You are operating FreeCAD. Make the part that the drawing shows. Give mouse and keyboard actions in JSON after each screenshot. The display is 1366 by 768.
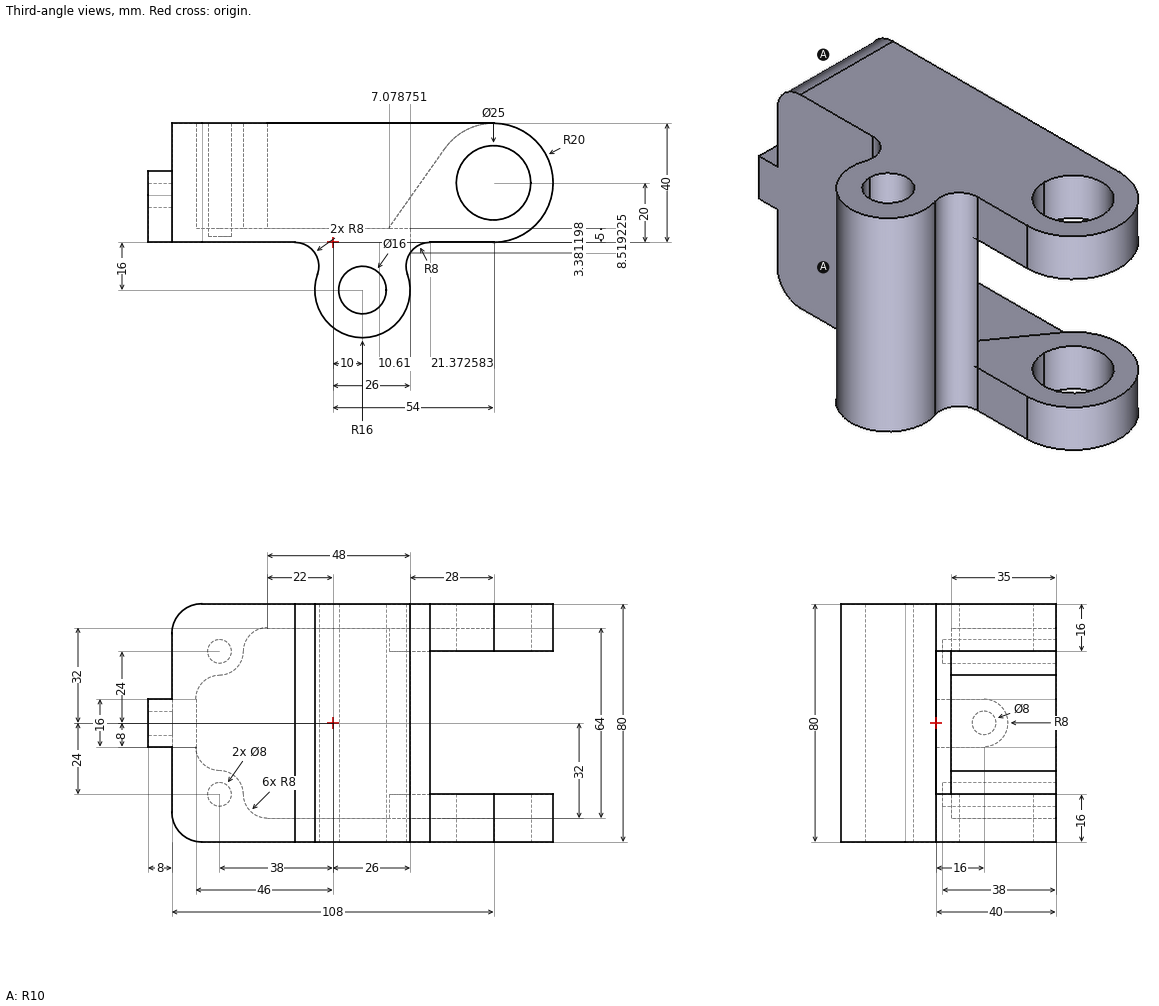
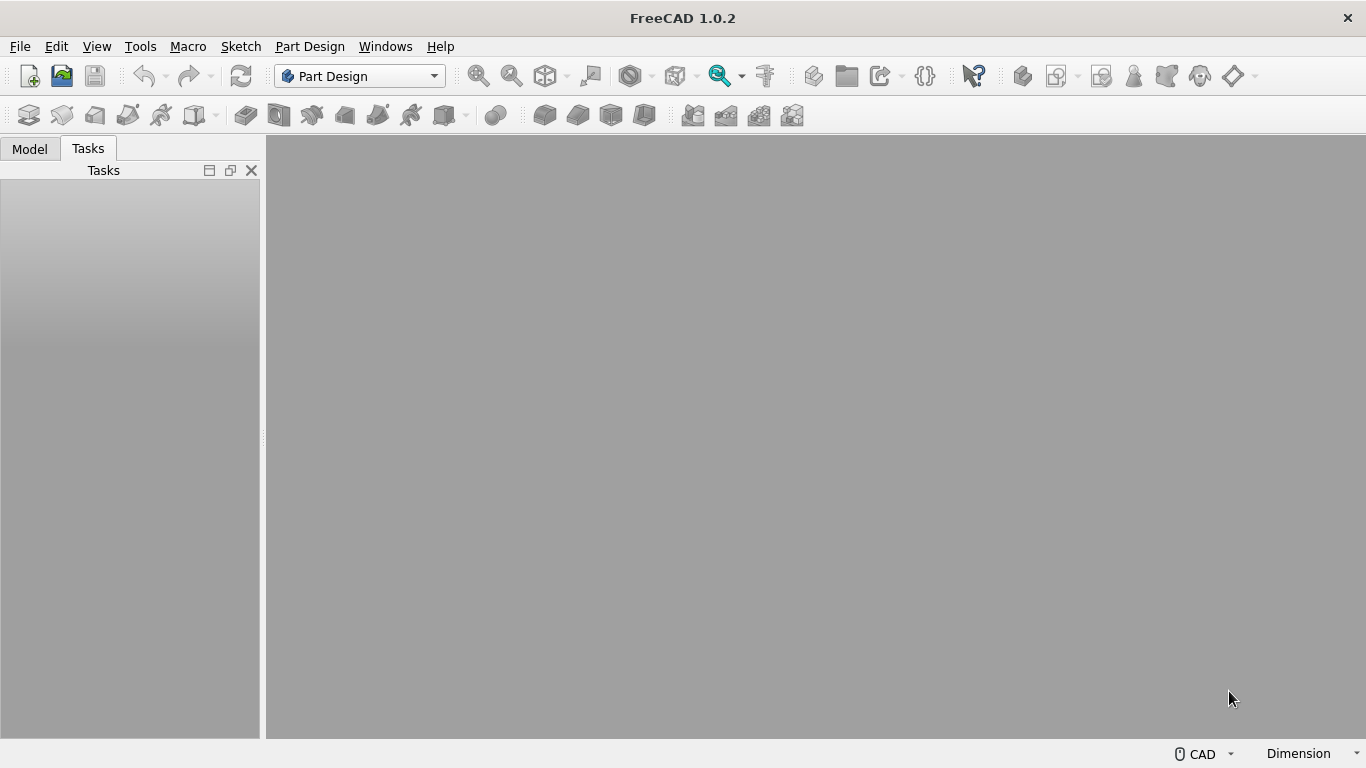
{"action": "left_click", "coordinate": [29, 76]}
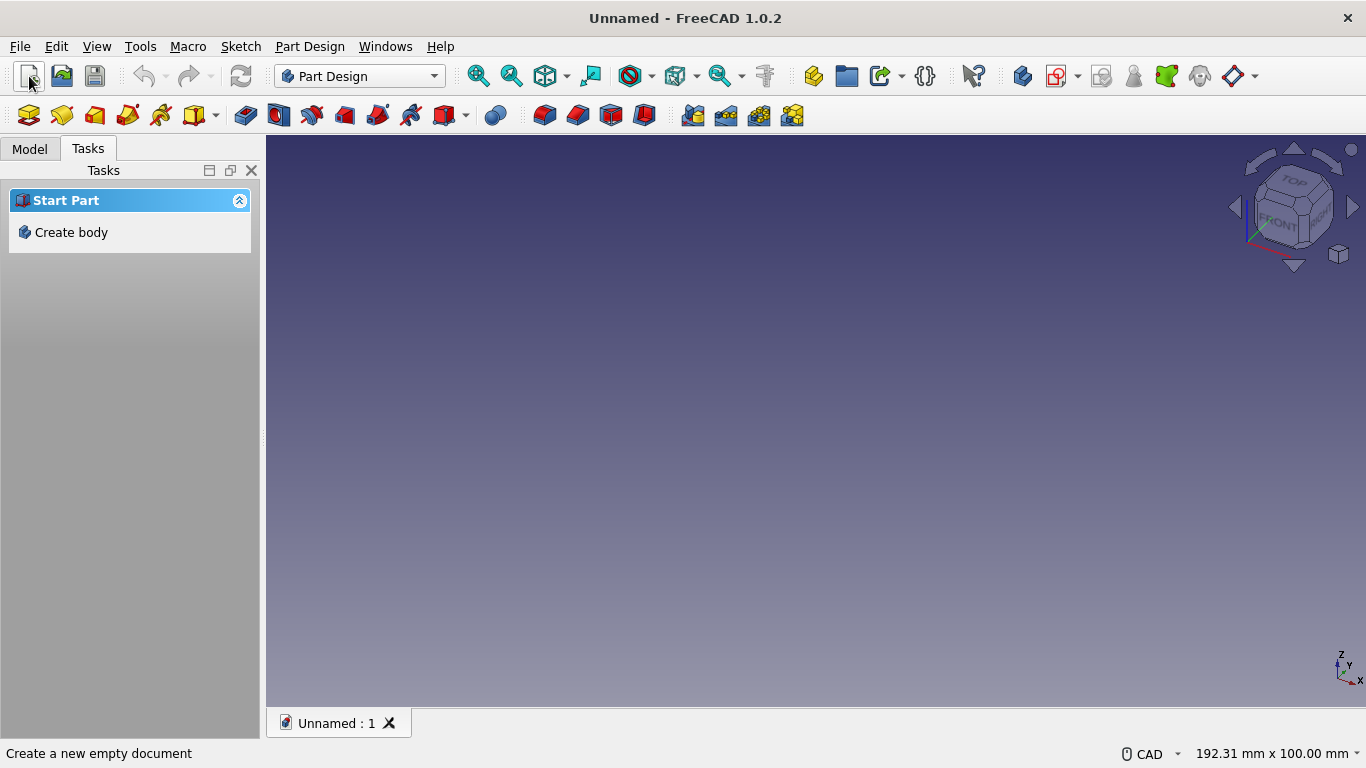
{"action": "left_click", "coordinate": [1056, 76]}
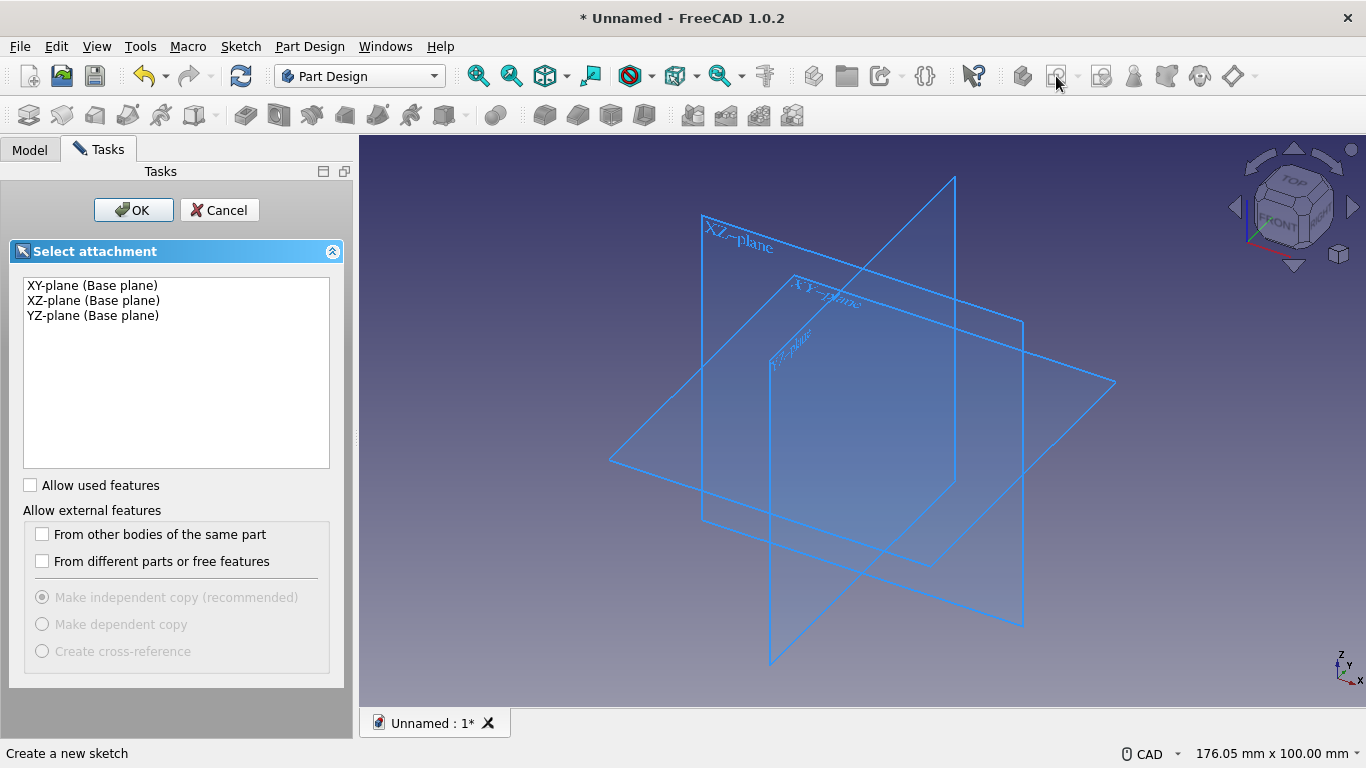
{"action": "left_click", "coordinate": [84, 300]}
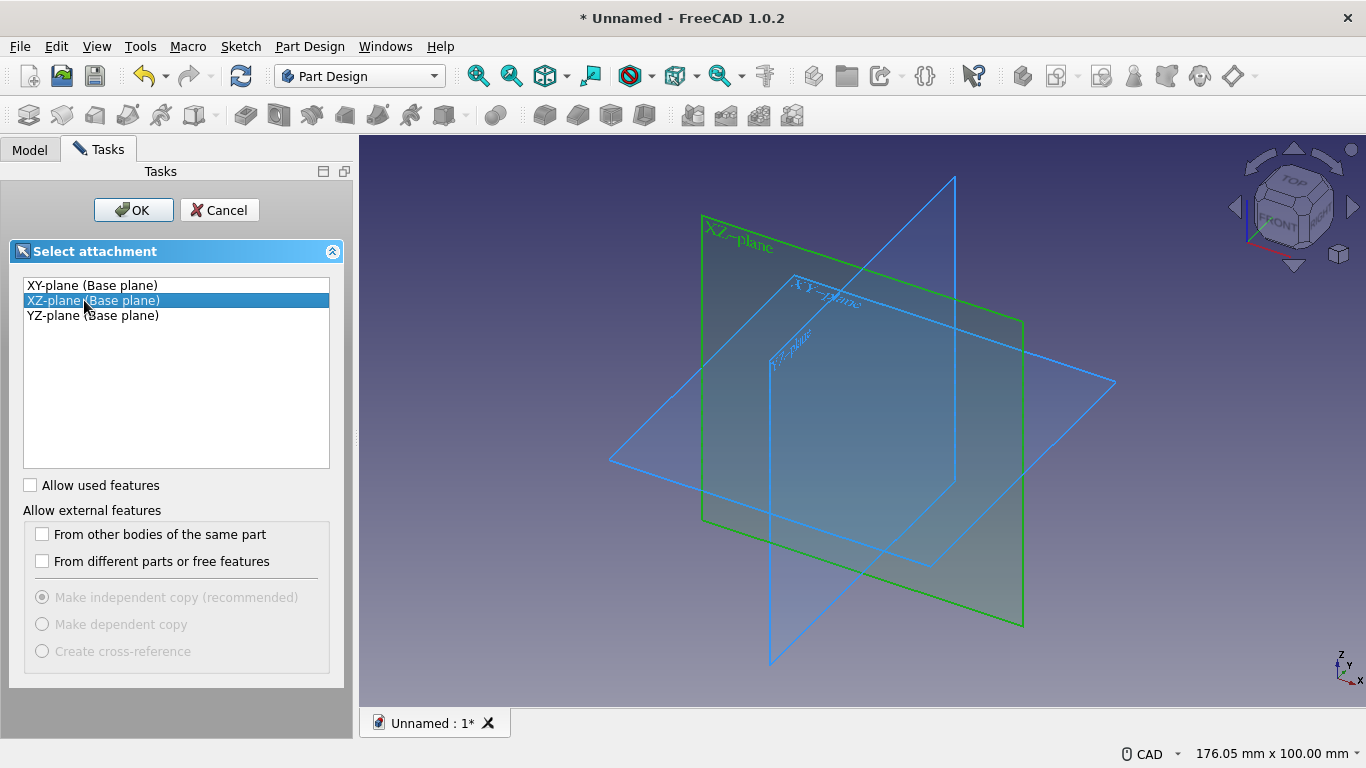
{"action": "left_click", "coordinate": [134, 210]}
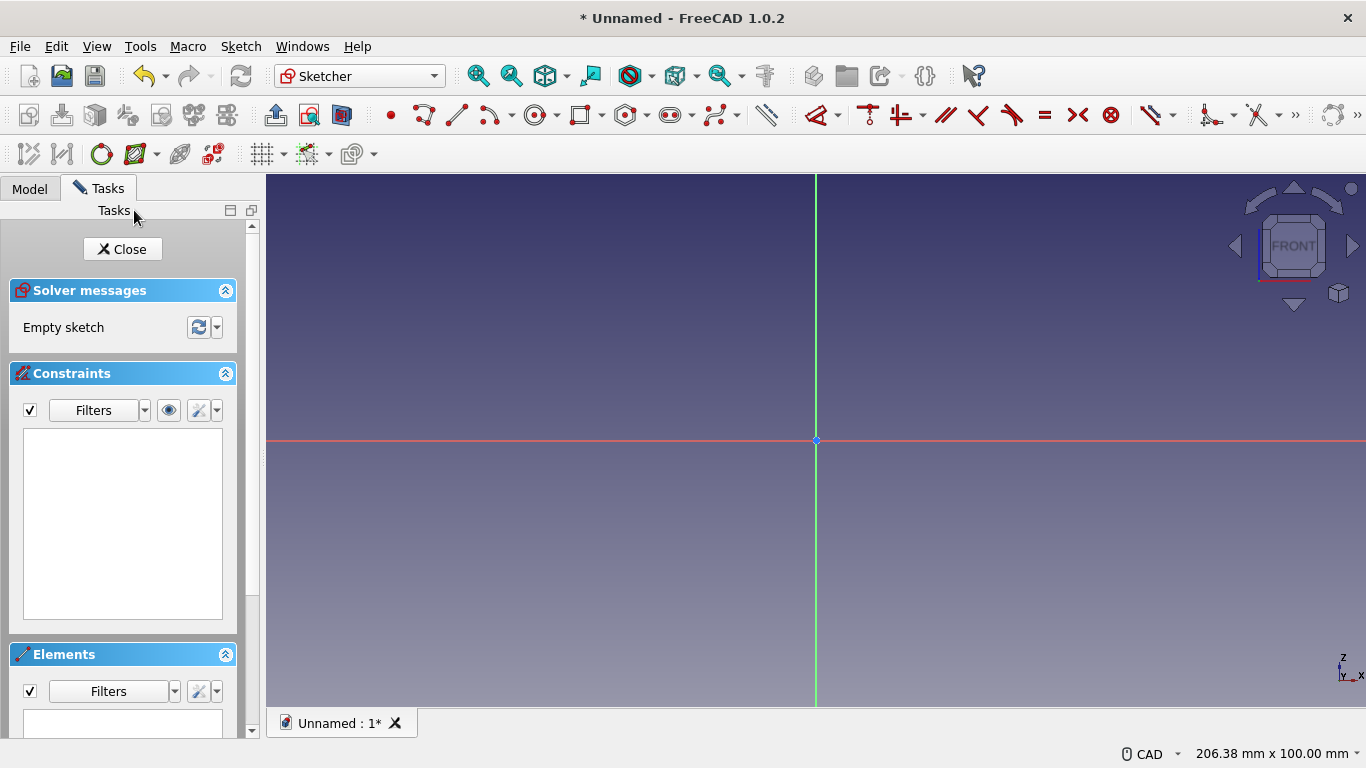
{"action": "key", "text": "g v"}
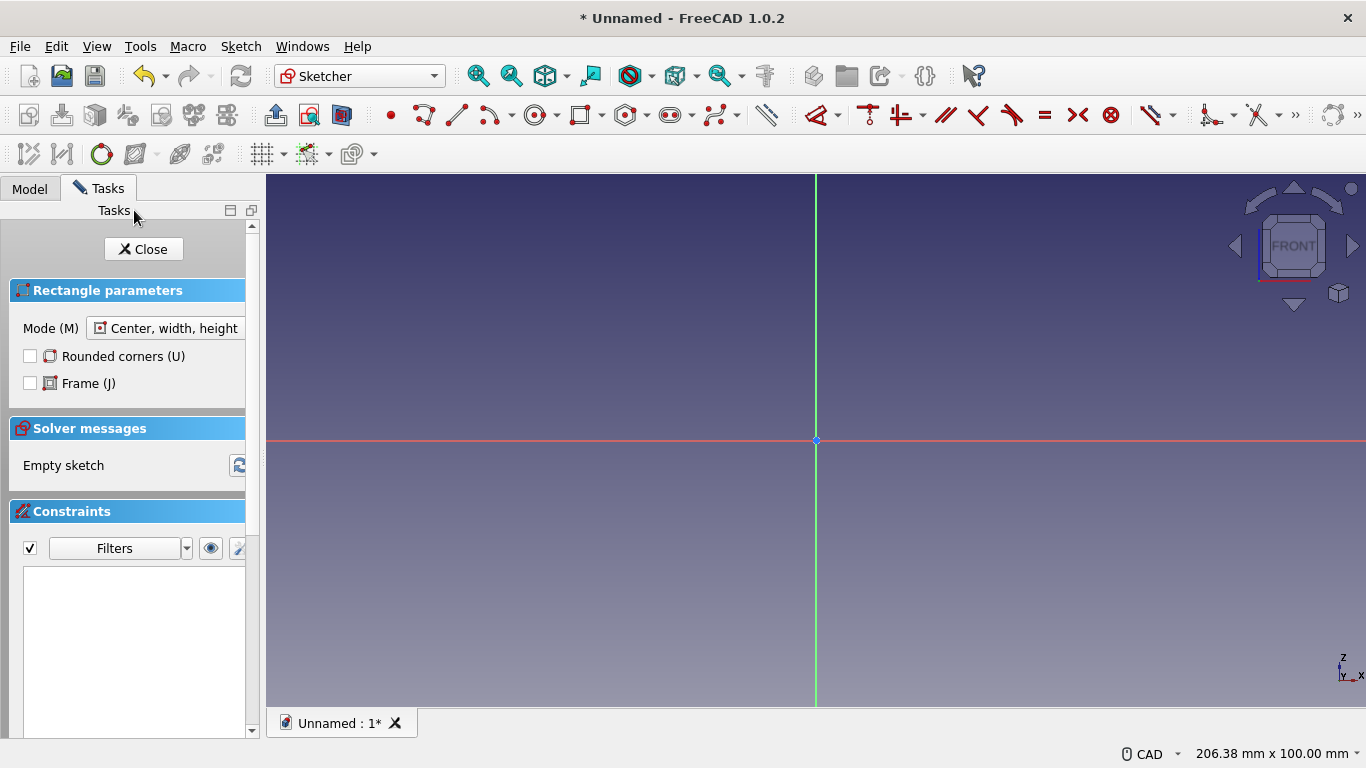
{"action": "left_click", "coordinate": [816, 440]}
{"action": "mouse_move", "coordinate": [1104, 227]}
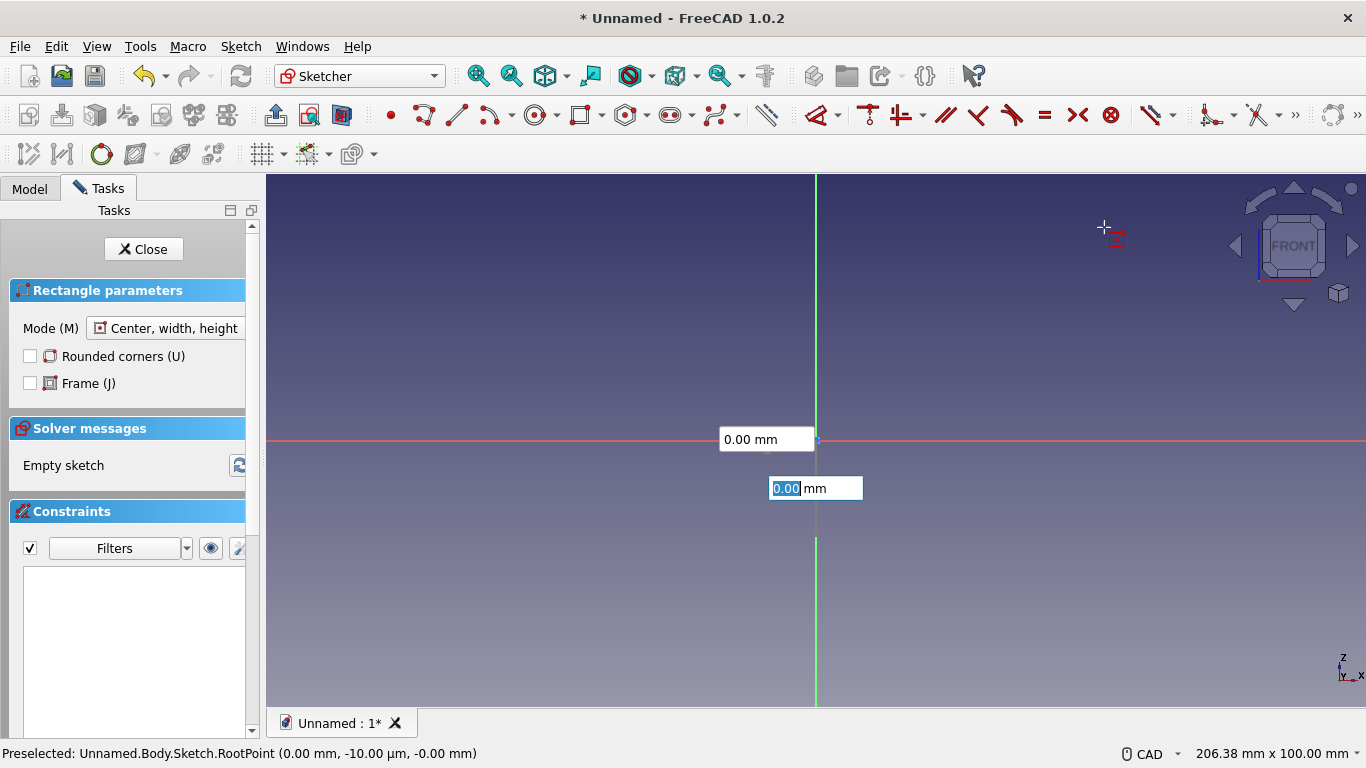
{"action": "type", "text": "108"}
{"action": "key", "text": "Tab"}
{"action": "type", "text": "80"}
{"action": "key", "text": "Return"}
{"action": "key", "text": "Escape"}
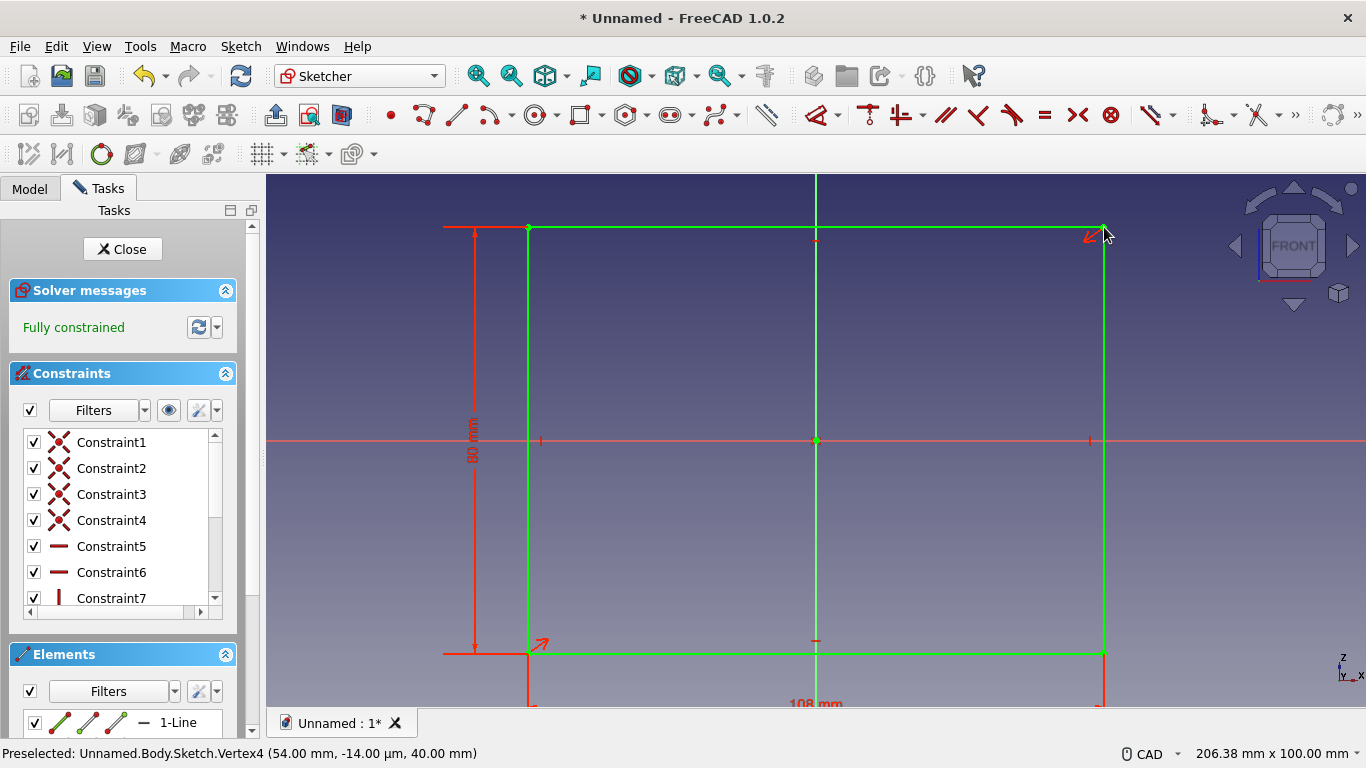
{"action": "left_click", "coordinate": [123, 249]}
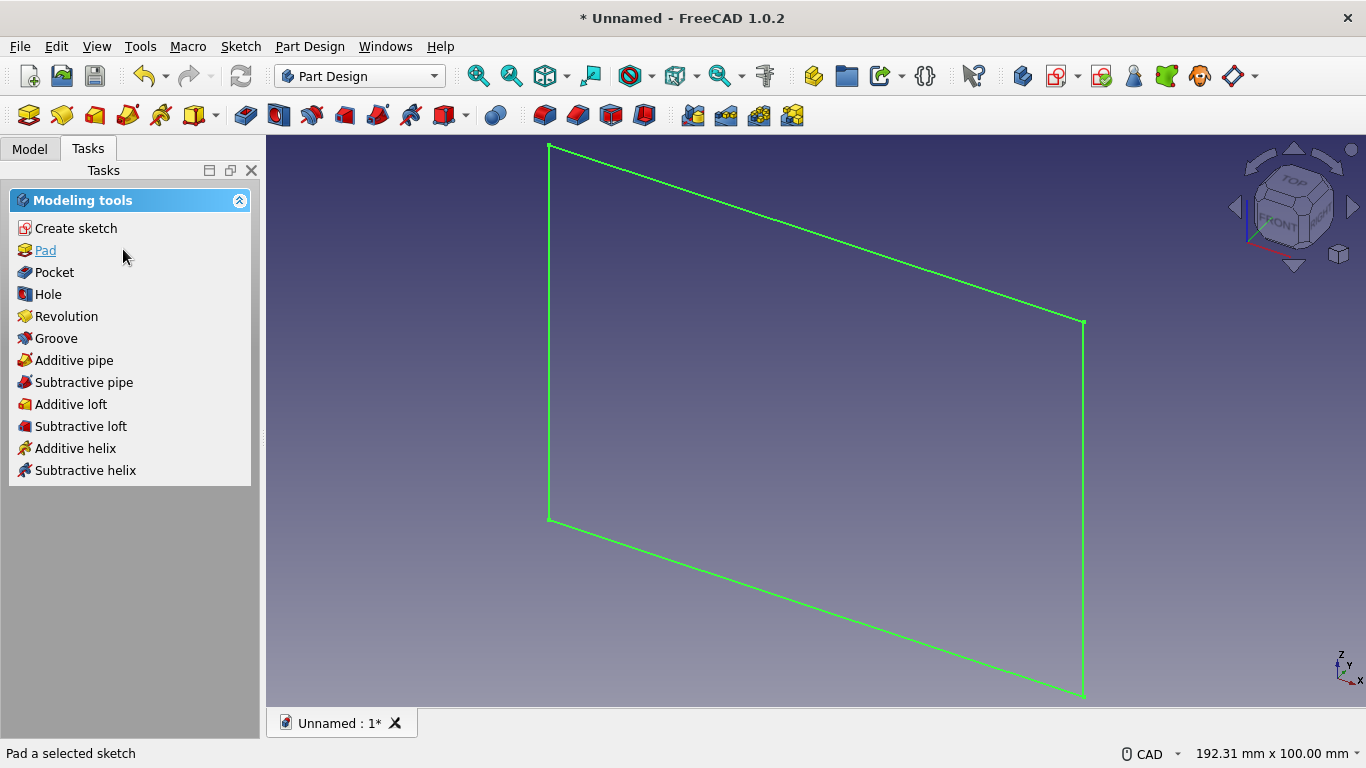
{"action": "left_click", "coordinate": [29, 116]}